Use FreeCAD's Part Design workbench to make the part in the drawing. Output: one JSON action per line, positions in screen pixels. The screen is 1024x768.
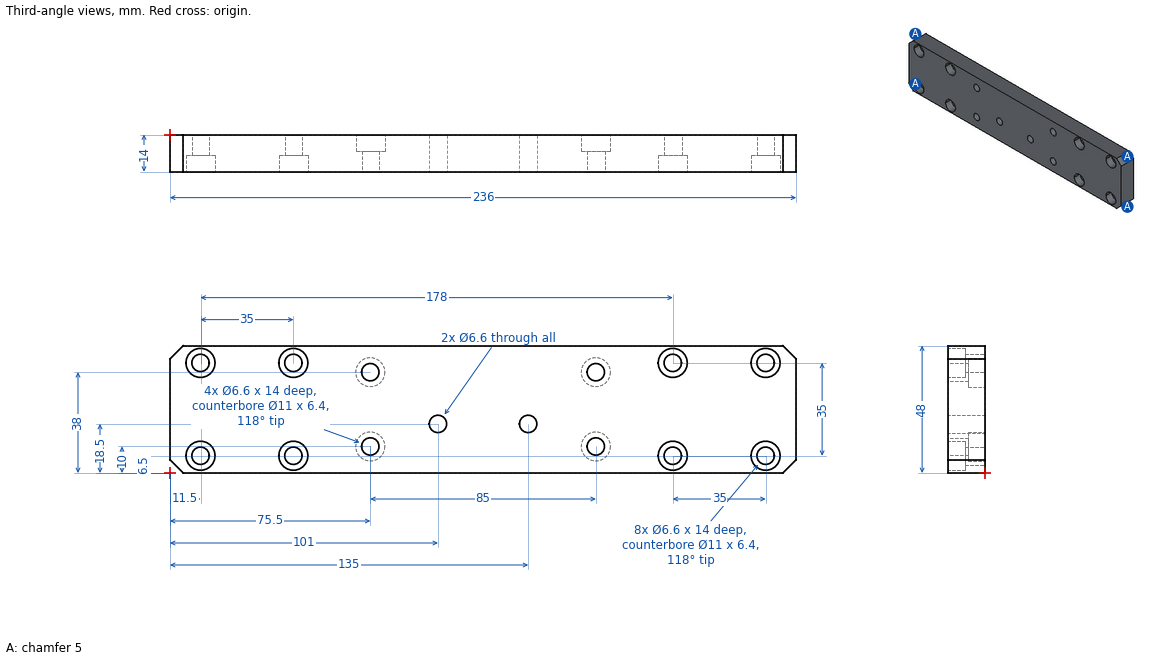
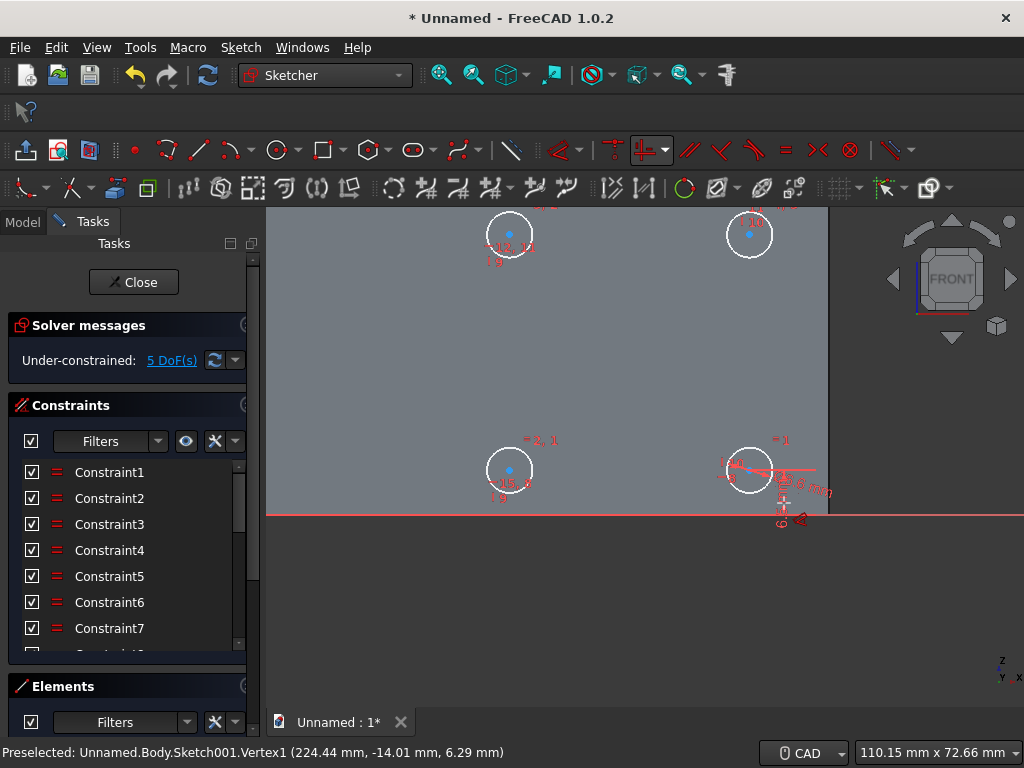
{"action": "scroll", "coordinate": [769, 488], "scroll_direction": "down", "scroll_amount": 7}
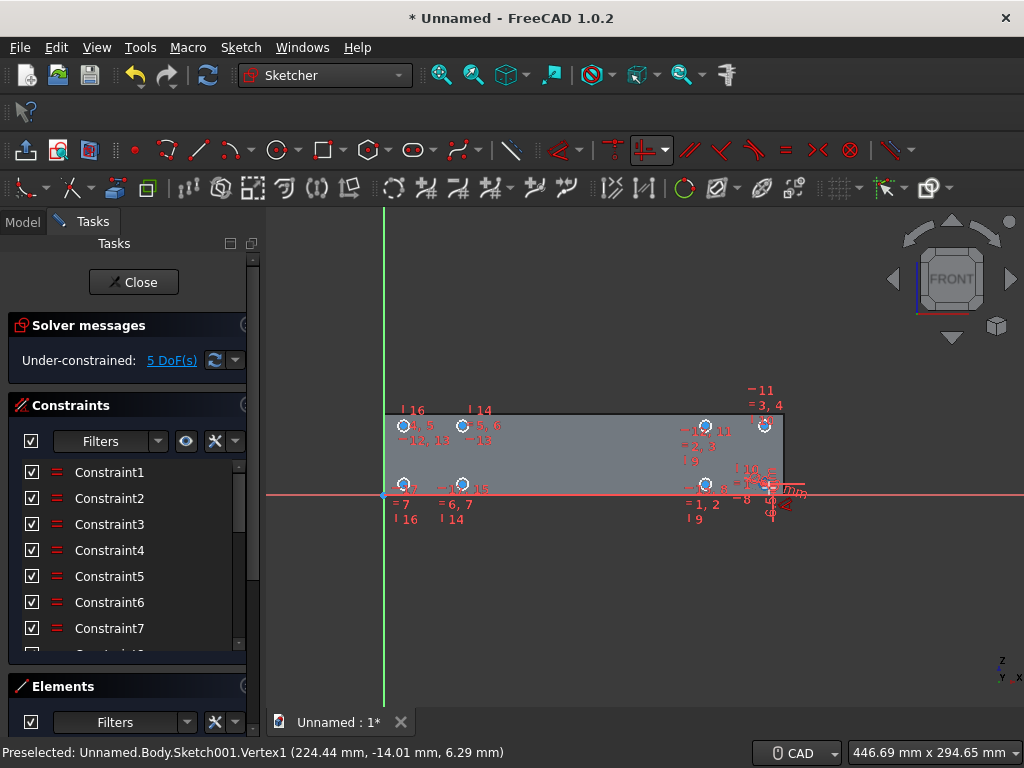
{"action": "left_click", "coordinate": [765, 484]}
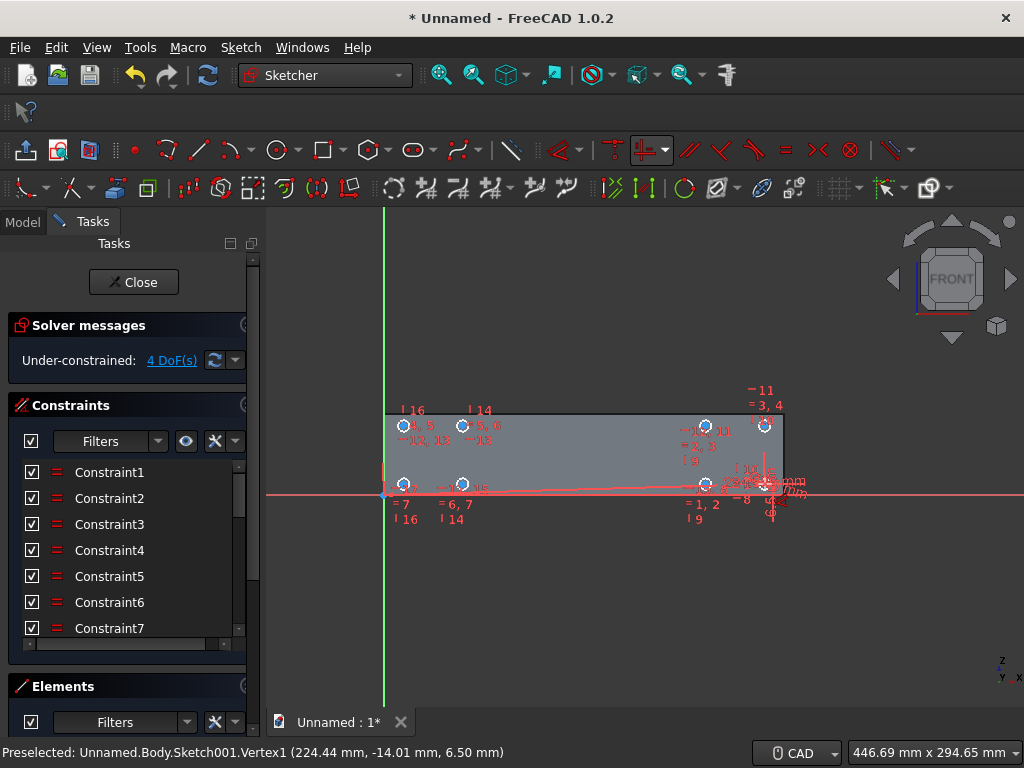
{"action": "left_click", "coordinate": [706, 484]}
{"action": "left_click", "coordinate": [735, 518]}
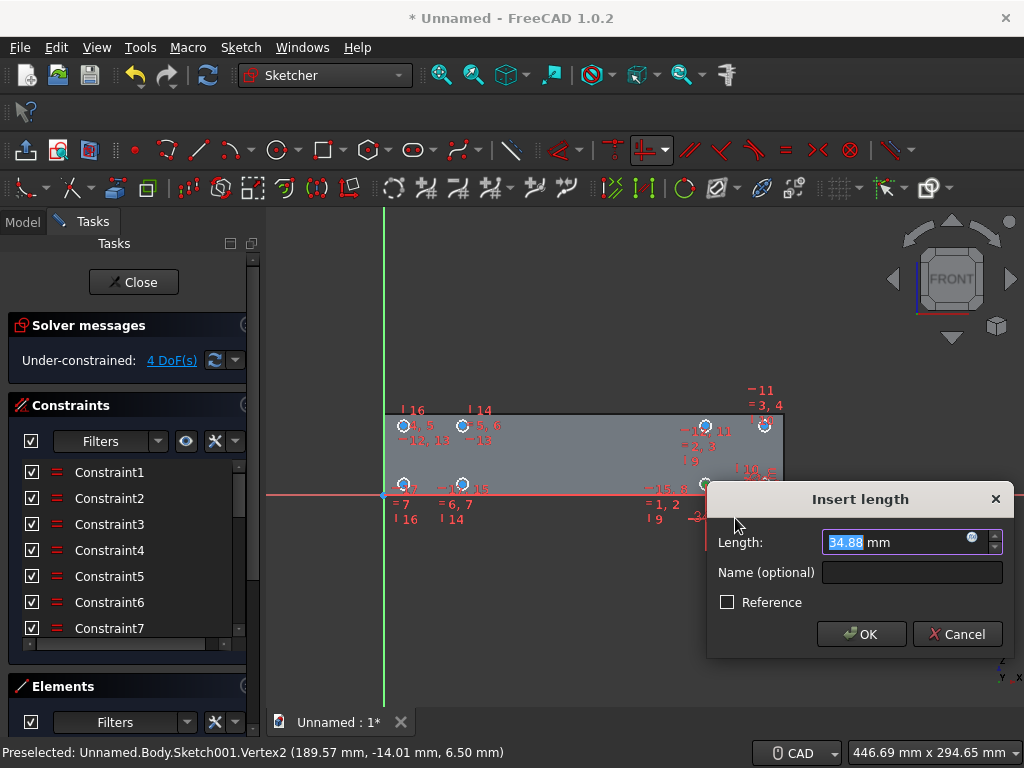
{"action": "type", "text": "35"}
{"action": "key", "text": "Return"}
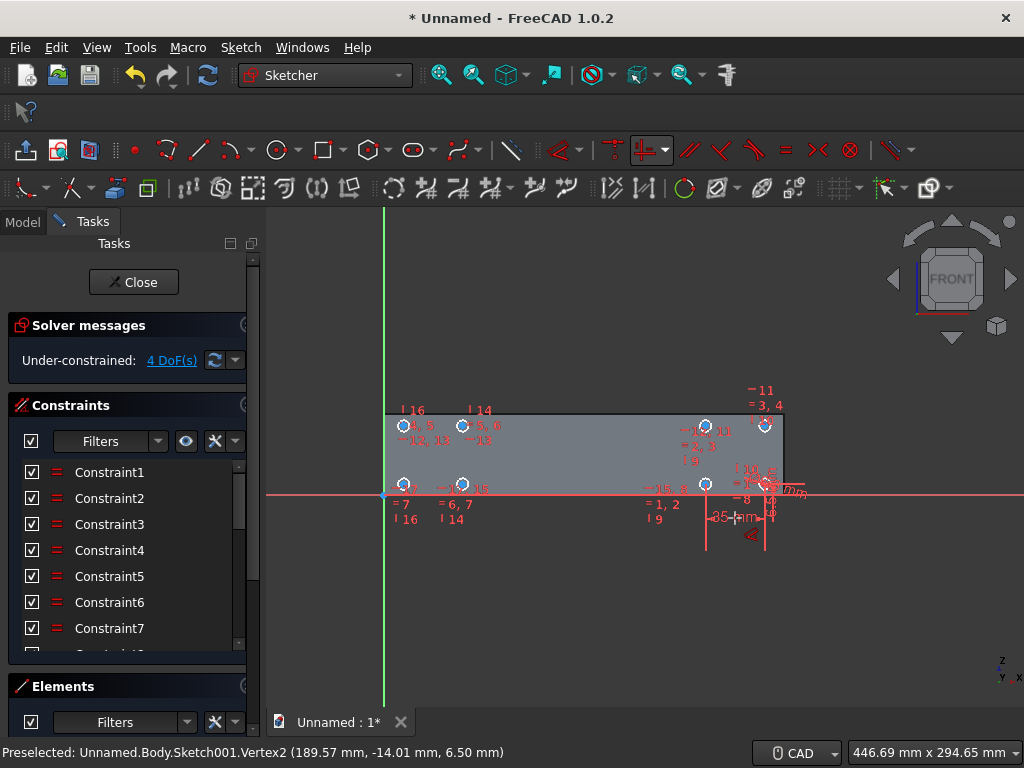
{"action": "left_click", "coordinate": [706, 484]}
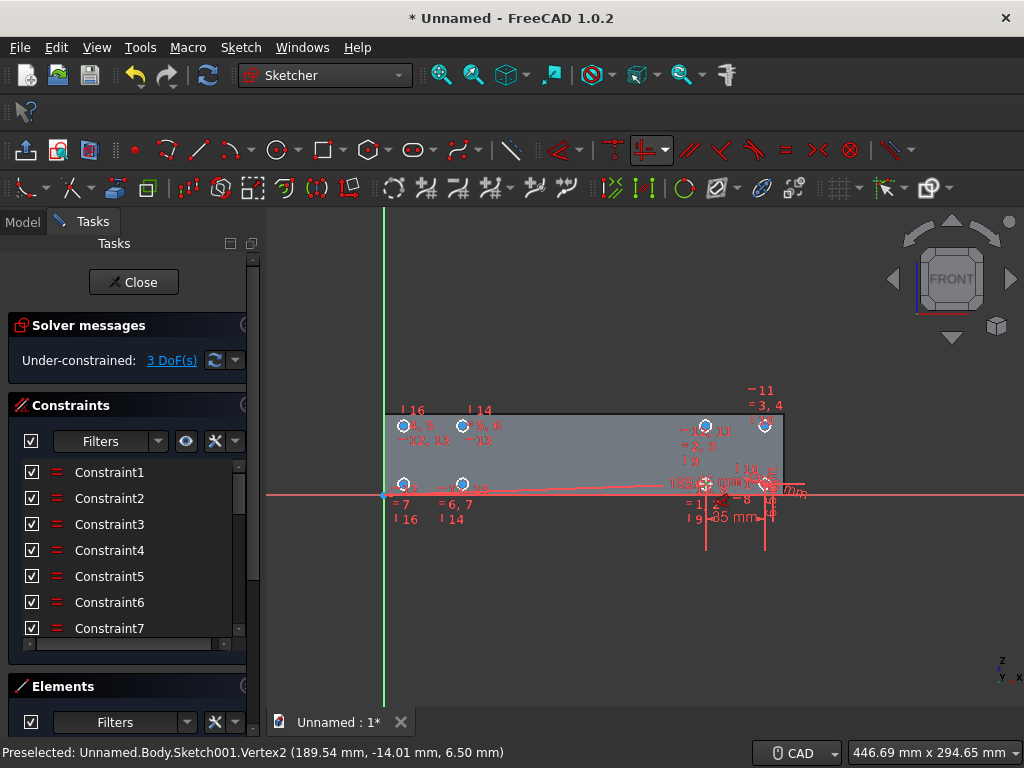
{"action": "left_click", "coordinate": [706, 426]}
{"action": "left_click", "coordinate": [740, 455]}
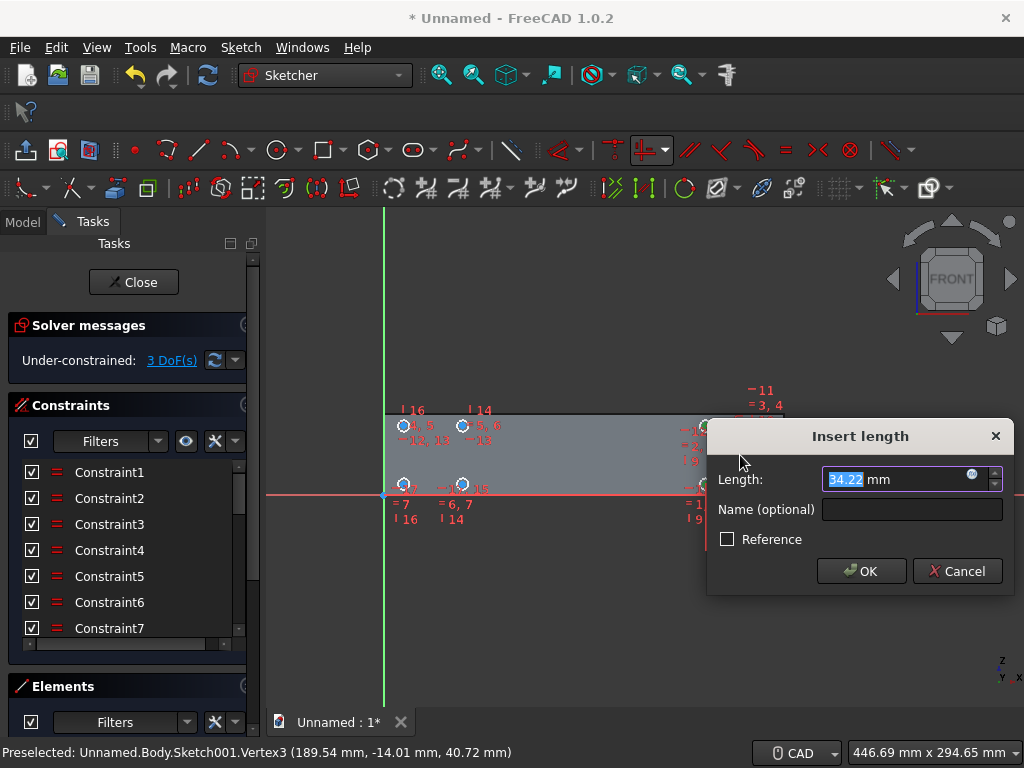
{"action": "type", "text": "35"}
{"action": "key", "text": "Return"}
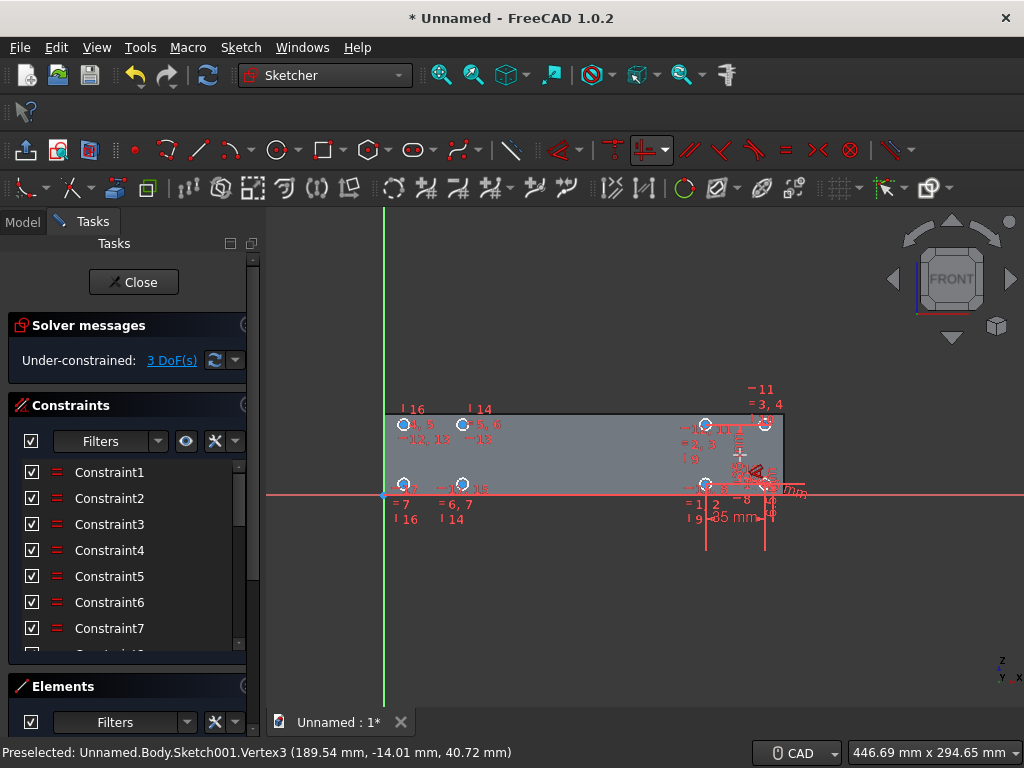
{"action": "left_click", "coordinate": [404, 425]}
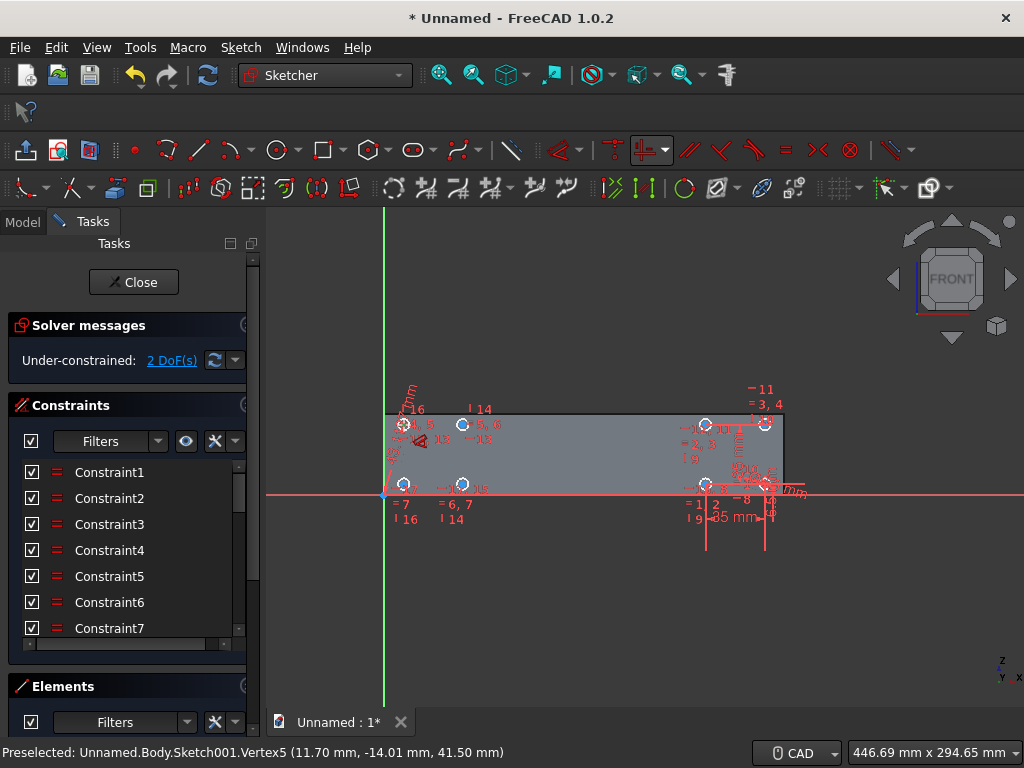
{"action": "left_click", "coordinate": [463, 425]}
{"action": "left_click", "coordinate": [433, 391]}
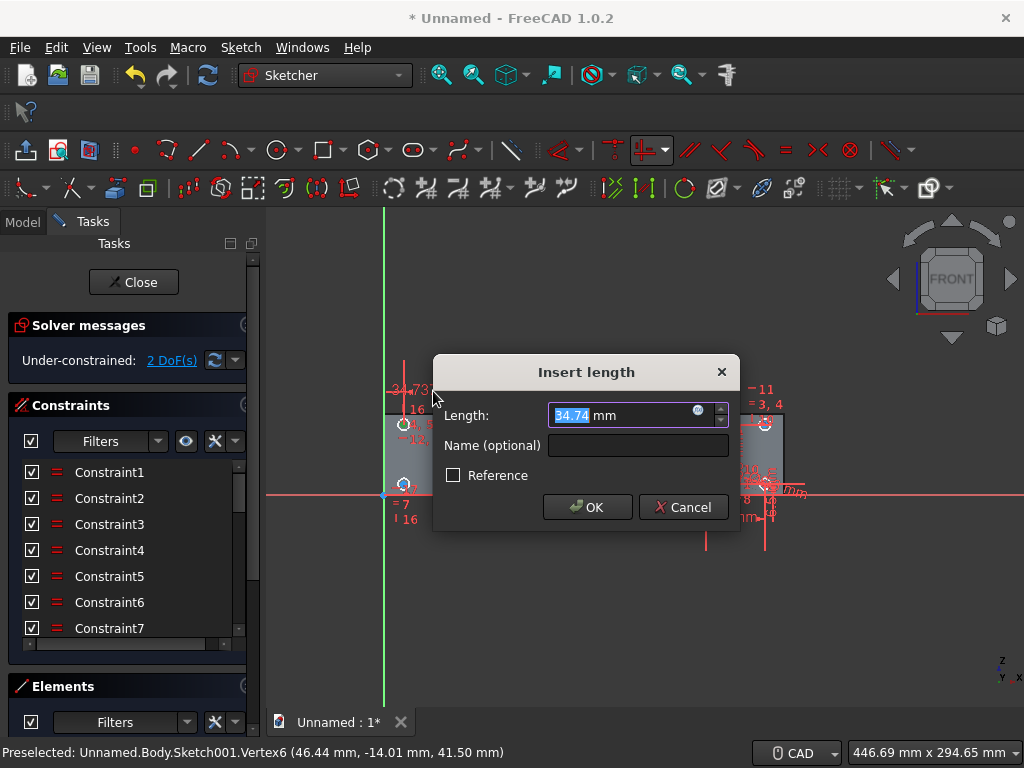
{"action": "type", "text": "35"}
{"action": "key", "text": "Return"}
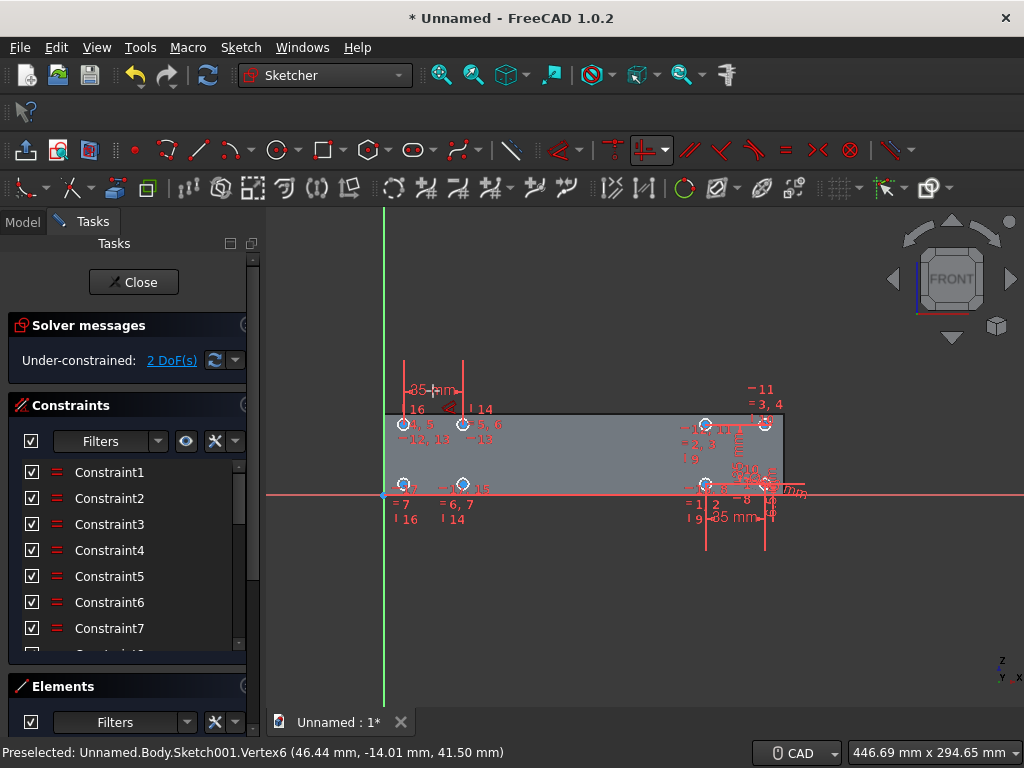
{"action": "scroll", "coordinate": [404, 425], "scroll_direction": "up", "scroll_amount": 4}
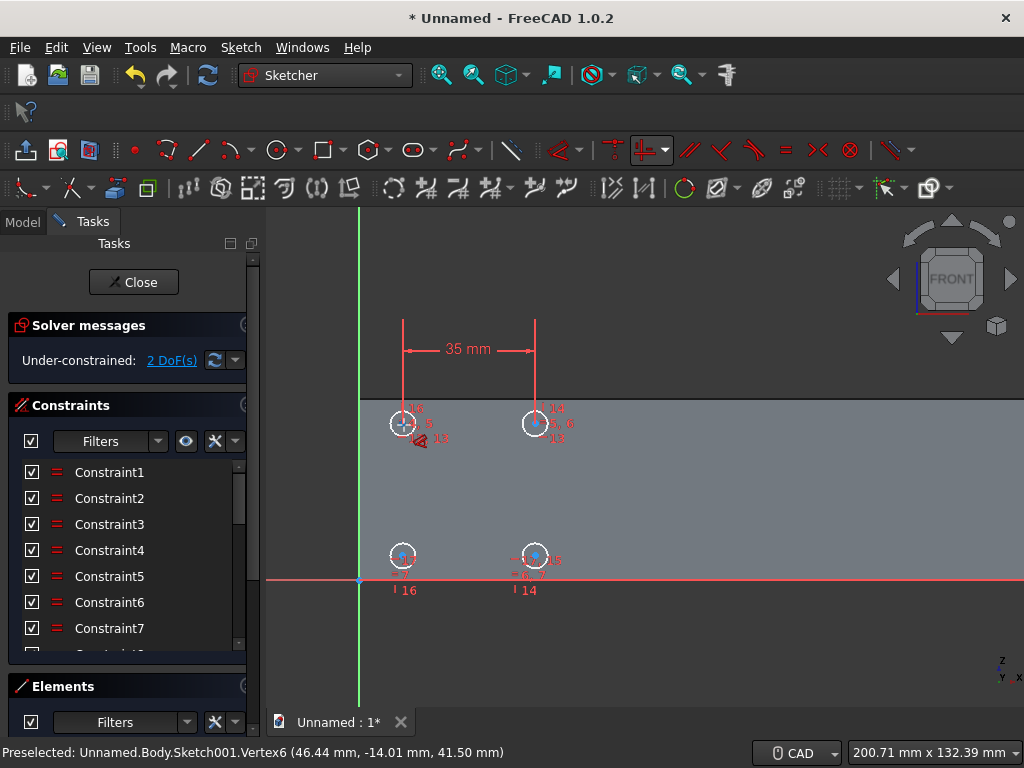
{"action": "left_click", "coordinate": [403, 424]}
{"action": "left_click", "coordinate": [381, 614]}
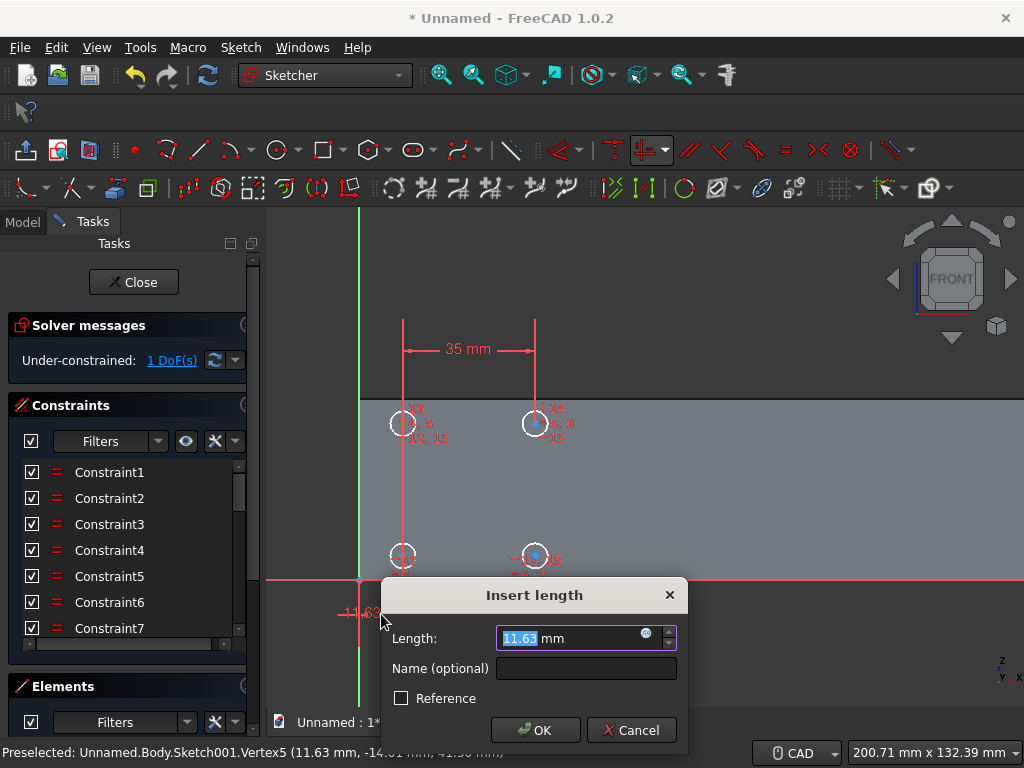
{"action": "type", "text": "11.5"}
{"action": "key", "text": "Return"}